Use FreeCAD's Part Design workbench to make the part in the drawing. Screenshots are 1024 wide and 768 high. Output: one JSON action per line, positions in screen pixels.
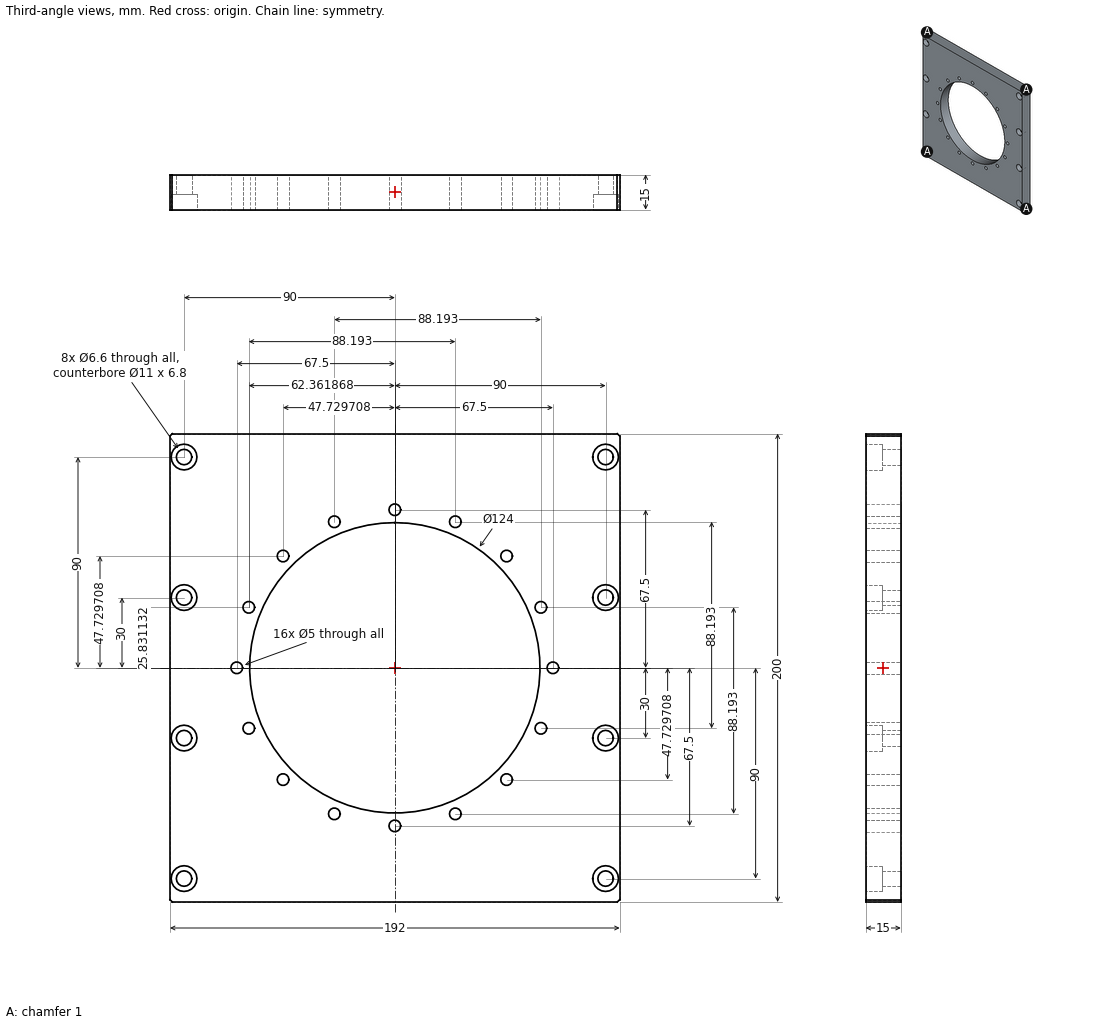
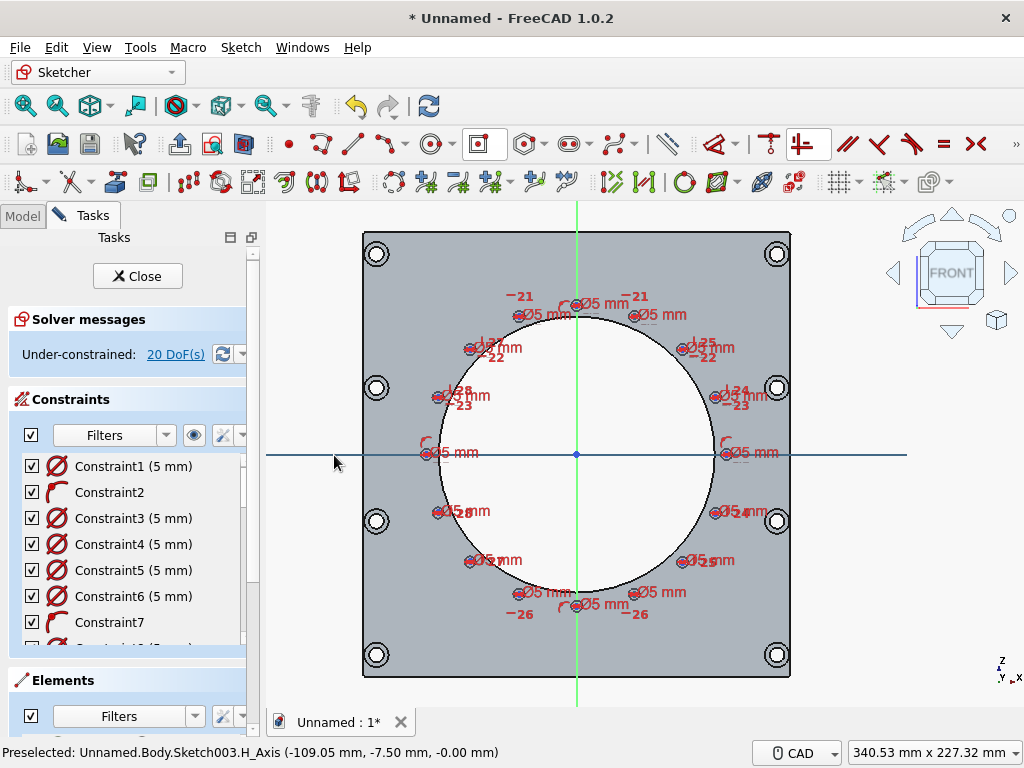
{"action": "left_click", "coordinate": [976, 144]}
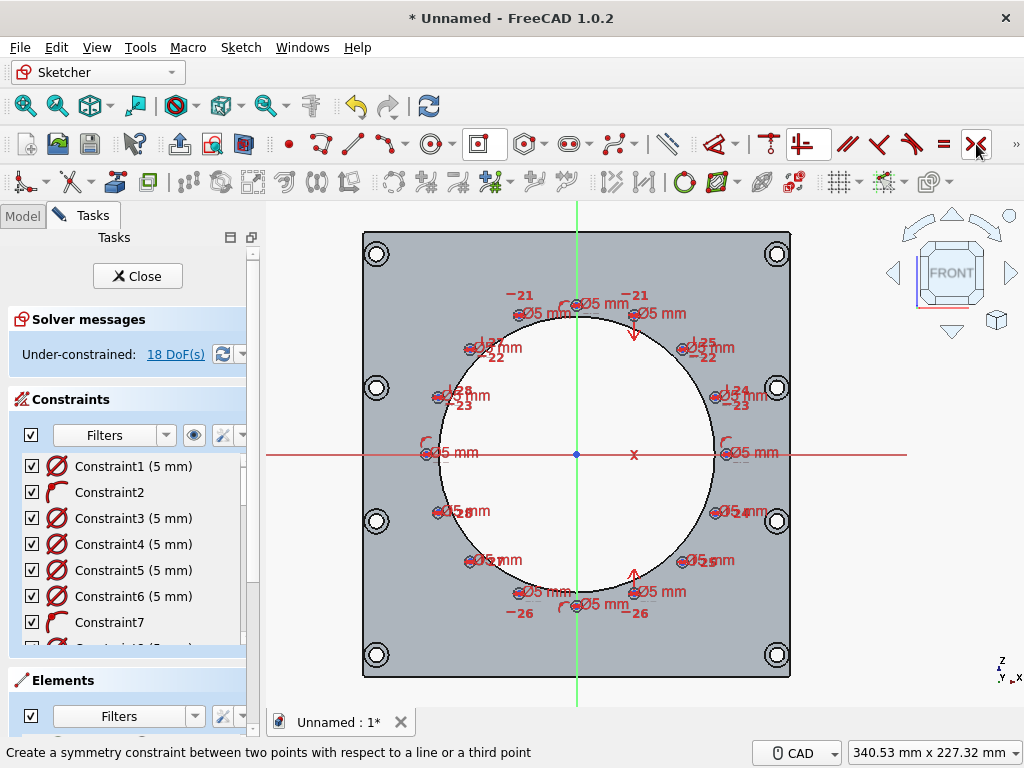
{"action": "left_click", "coordinate": [683, 562]}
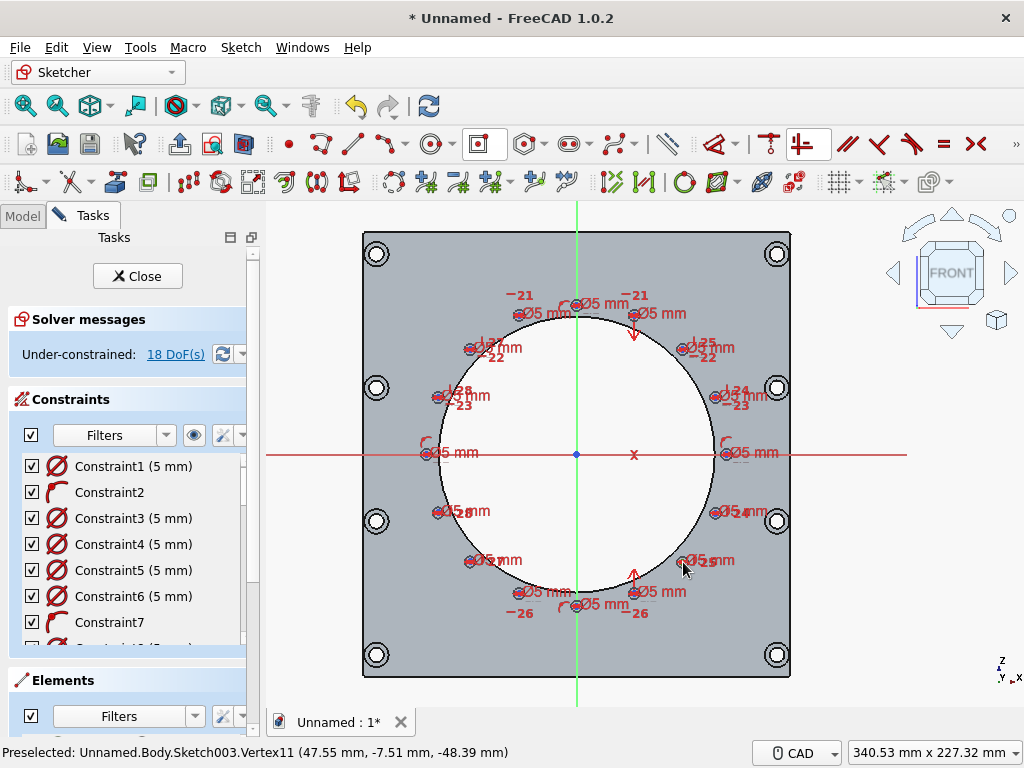
{"action": "left_click", "coordinate": [470, 562]}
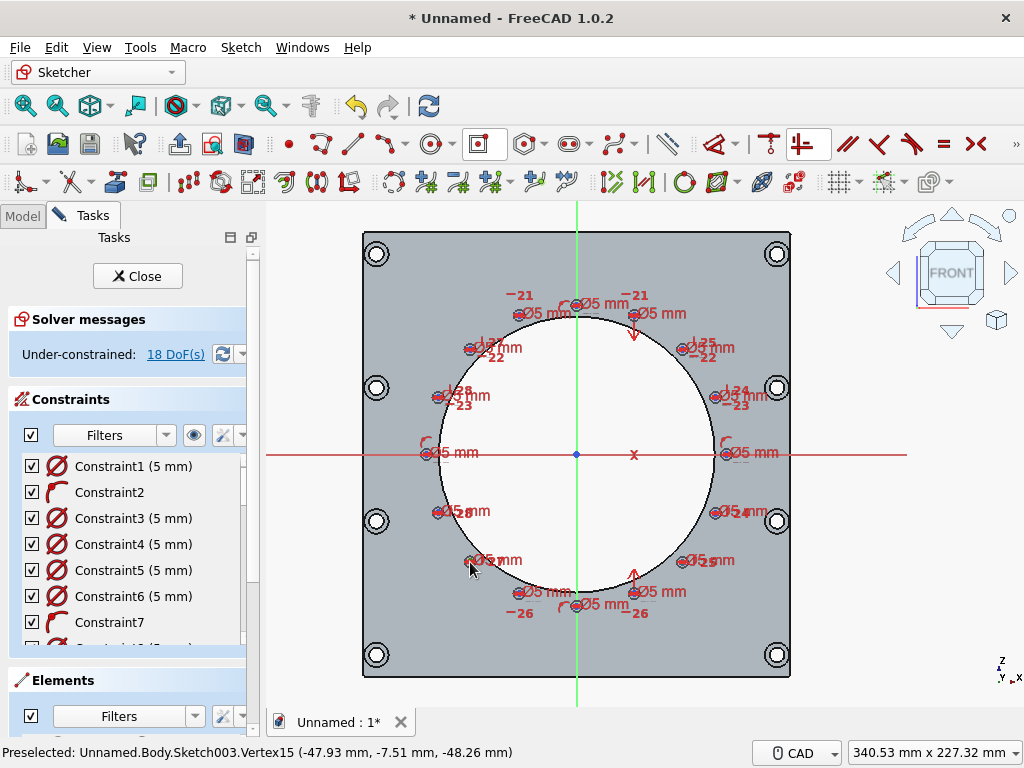
{"action": "left_click", "coordinate": [577, 647]}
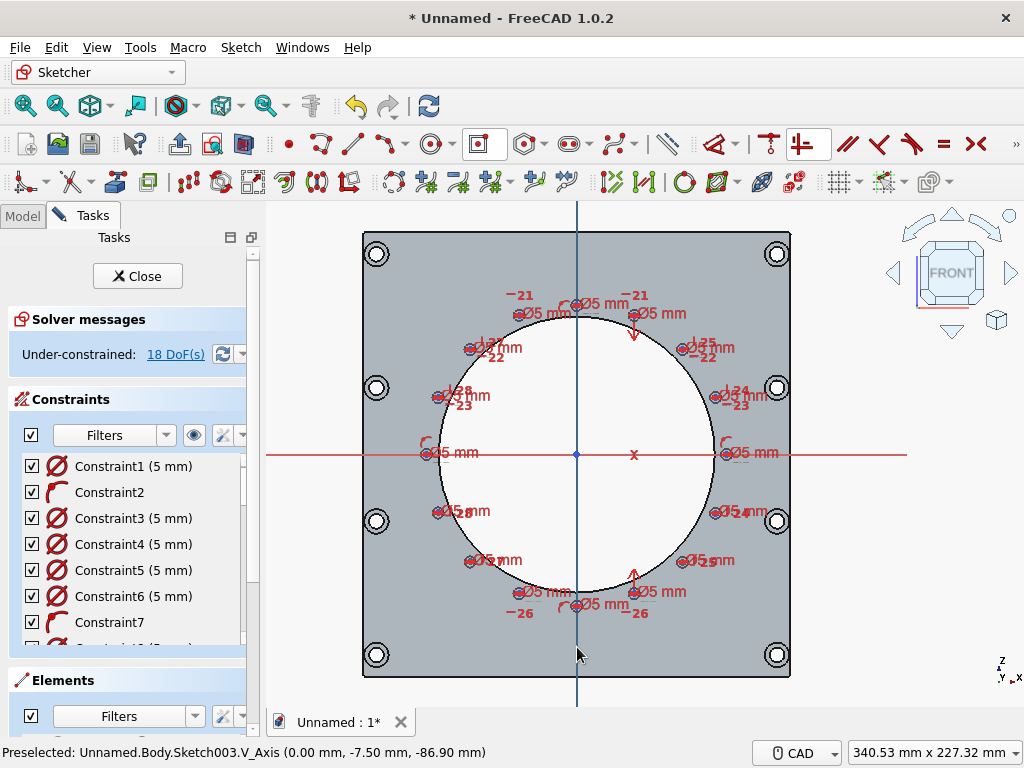
{"action": "left_click", "coordinate": [976, 144]}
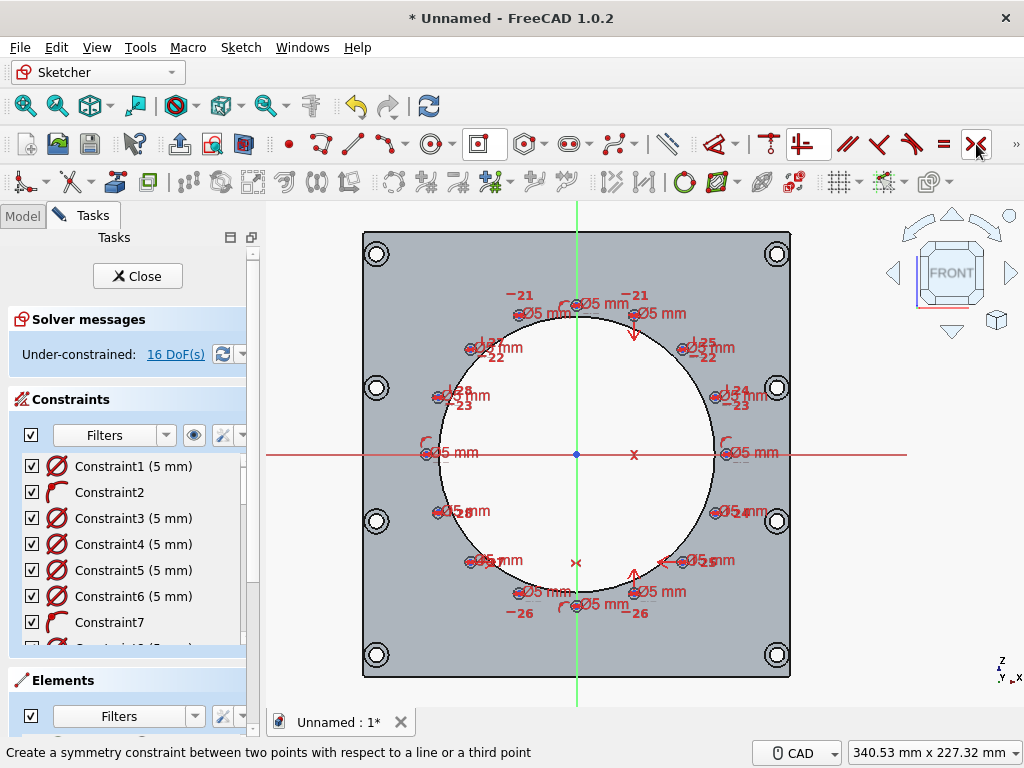
{"action": "left_click", "coordinate": [716, 513]}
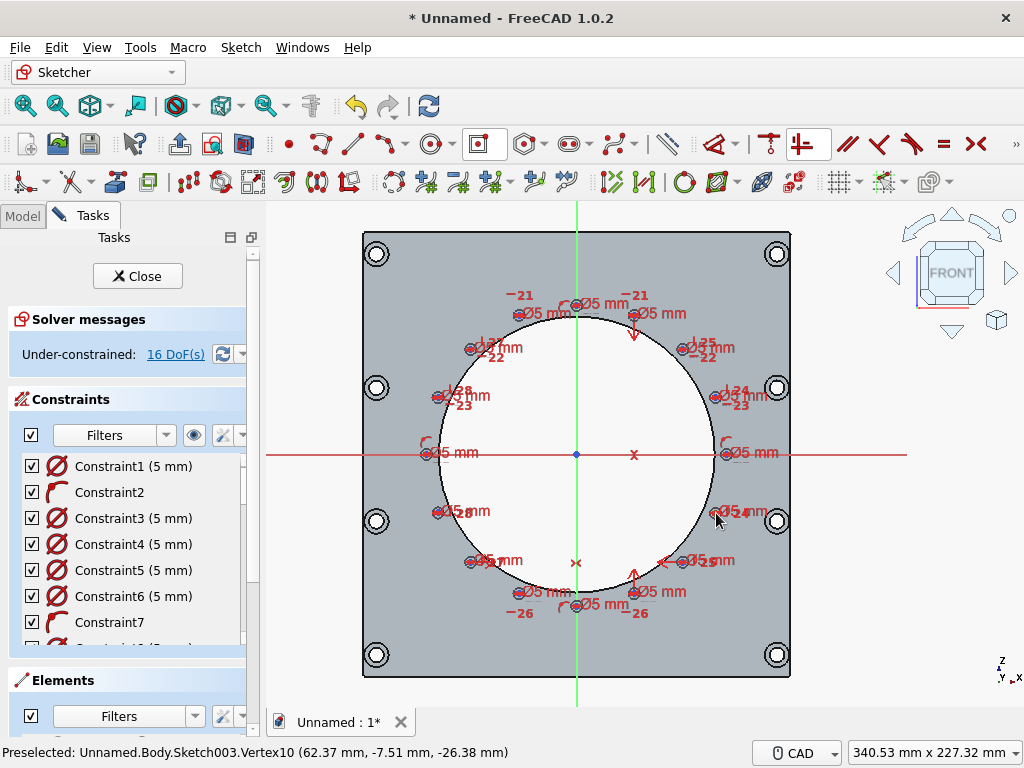
{"action": "left_click", "coordinate": [438, 513]}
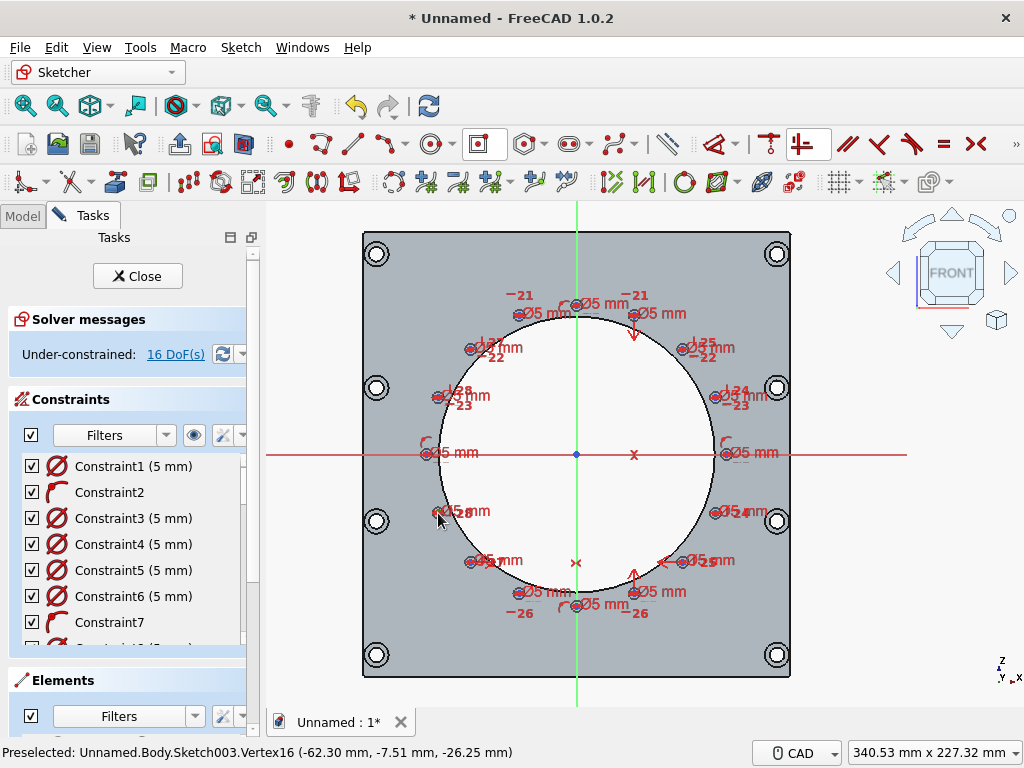
{"action": "left_click", "coordinate": [577, 647]}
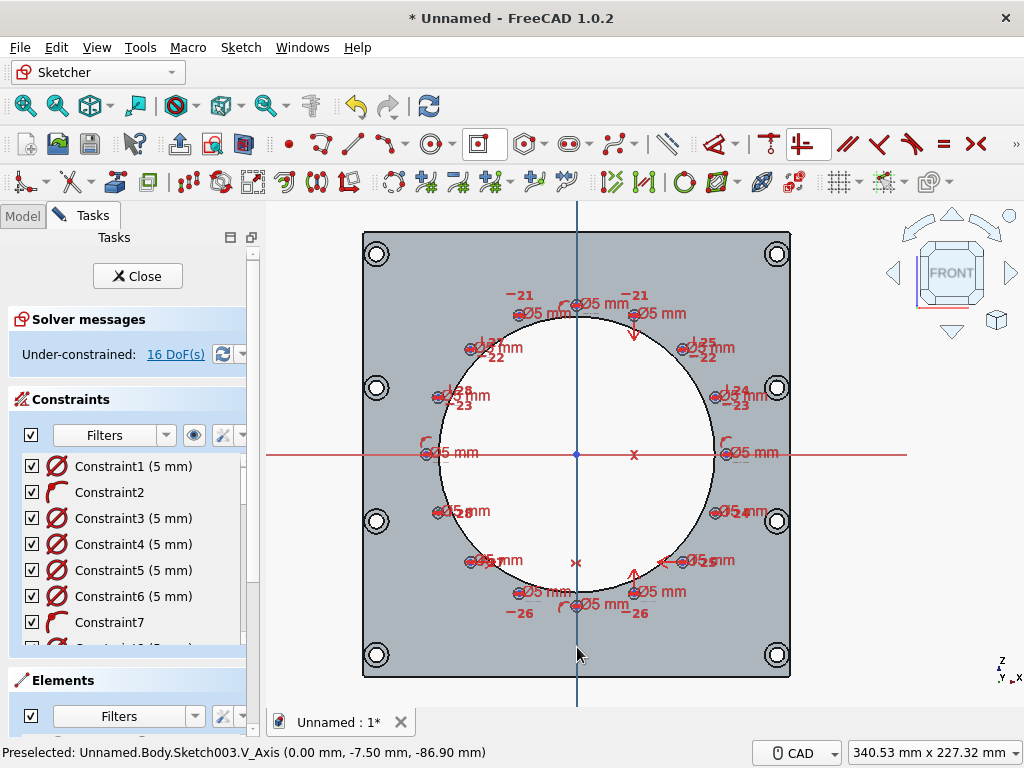
{"action": "left_click", "coordinate": [976, 144]}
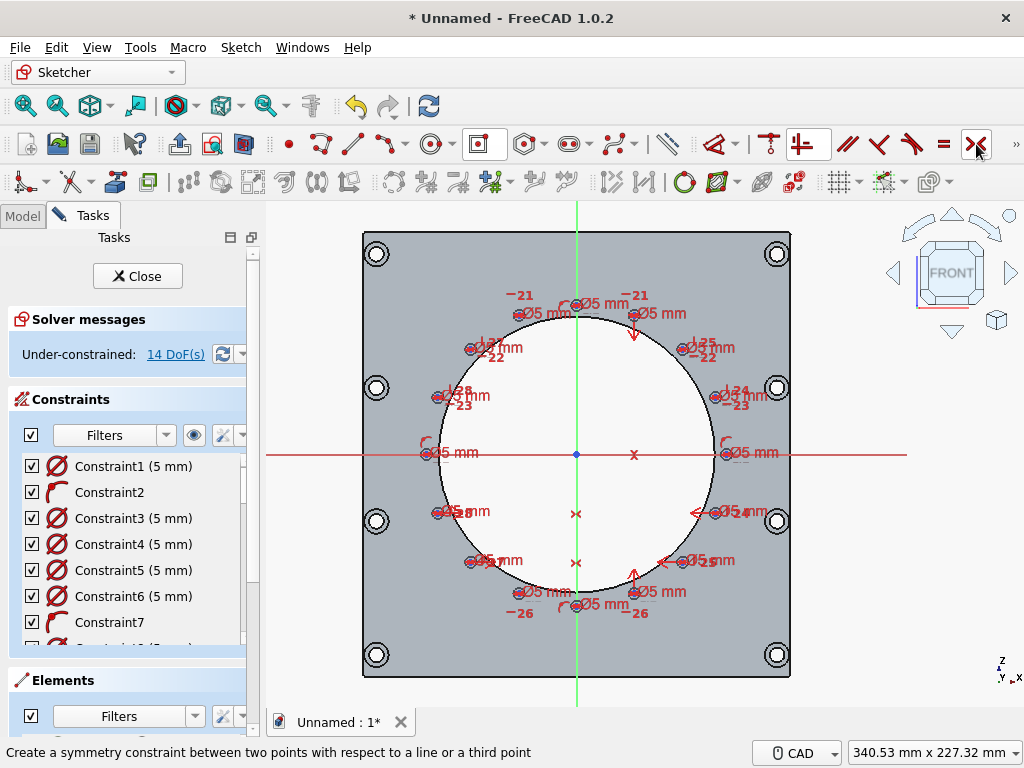
{"action": "left_click", "coordinate": [714, 144]}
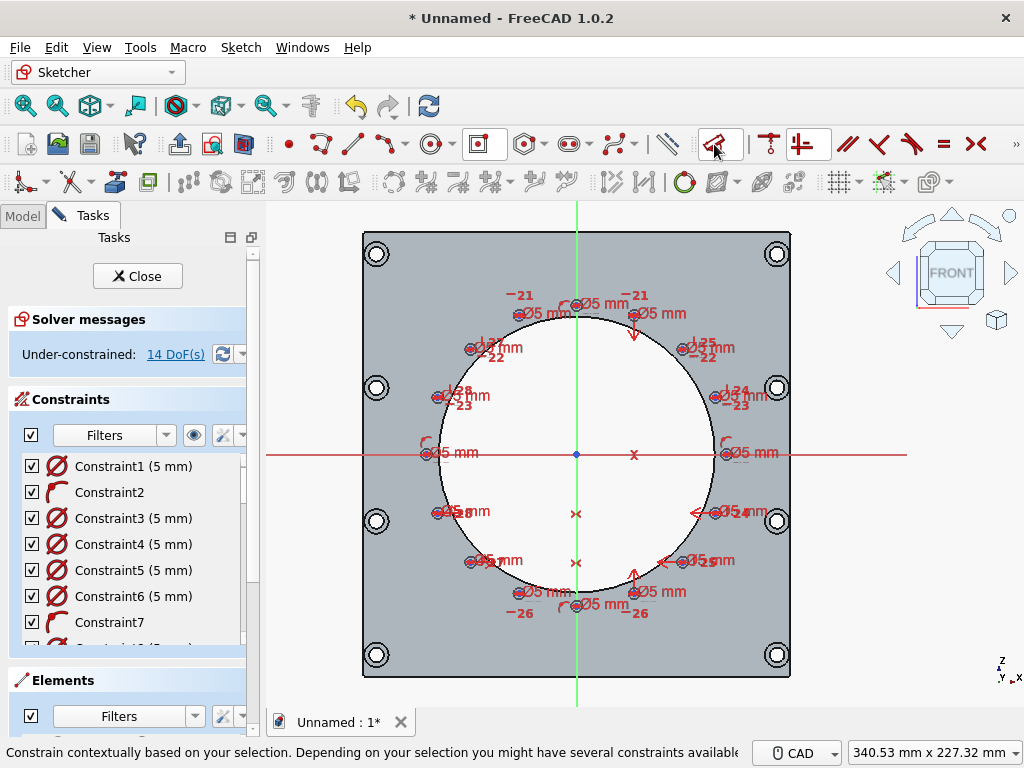
{"action": "left_click", "coordinate": [426, 455]}
{"action": "left_click", "coordinate": [502, 489]}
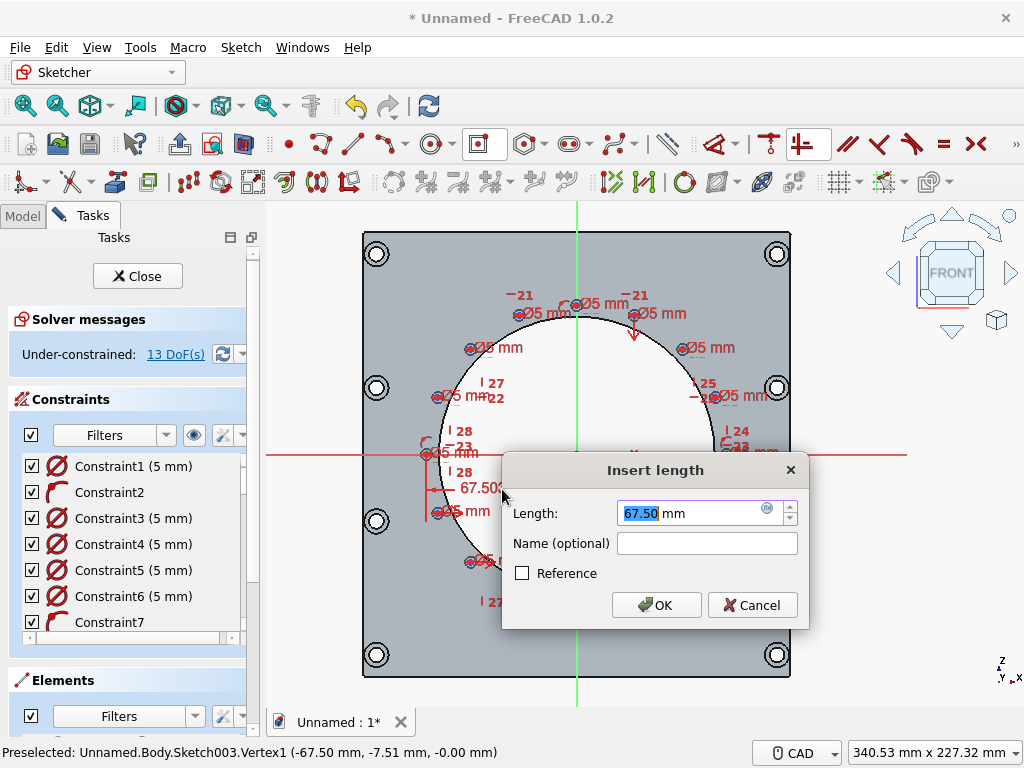
{"action": "type", "text": "67.5"}
{"action": "key", "text": "Return"}